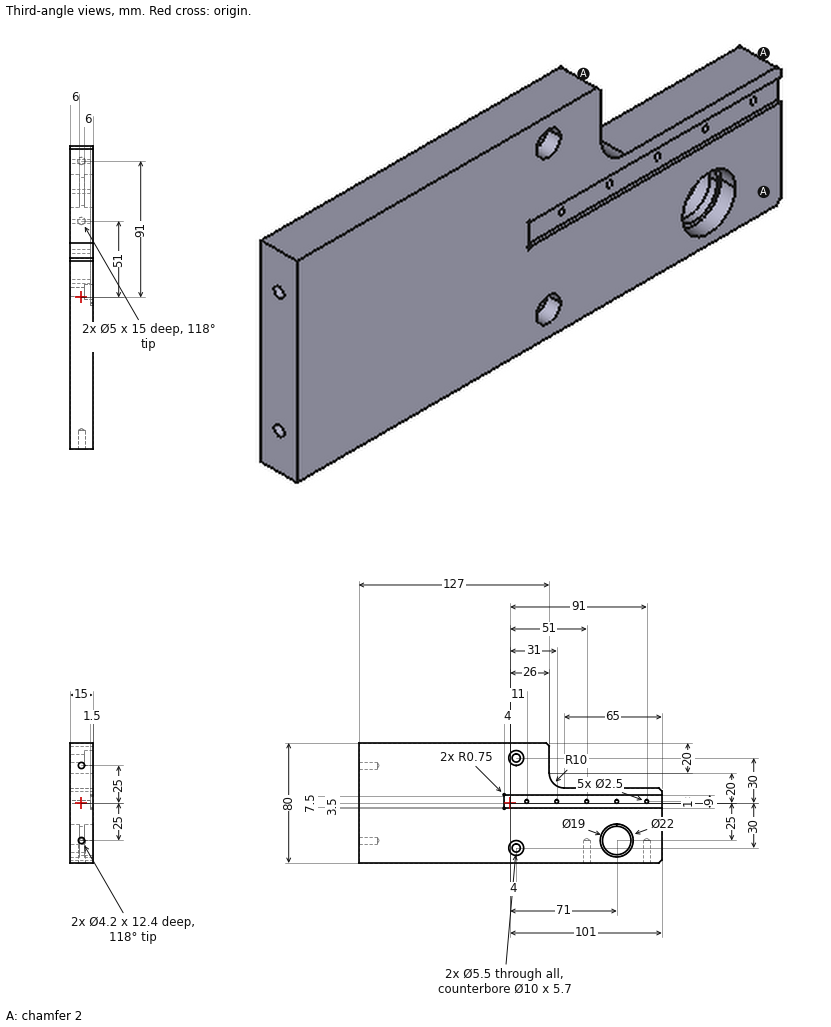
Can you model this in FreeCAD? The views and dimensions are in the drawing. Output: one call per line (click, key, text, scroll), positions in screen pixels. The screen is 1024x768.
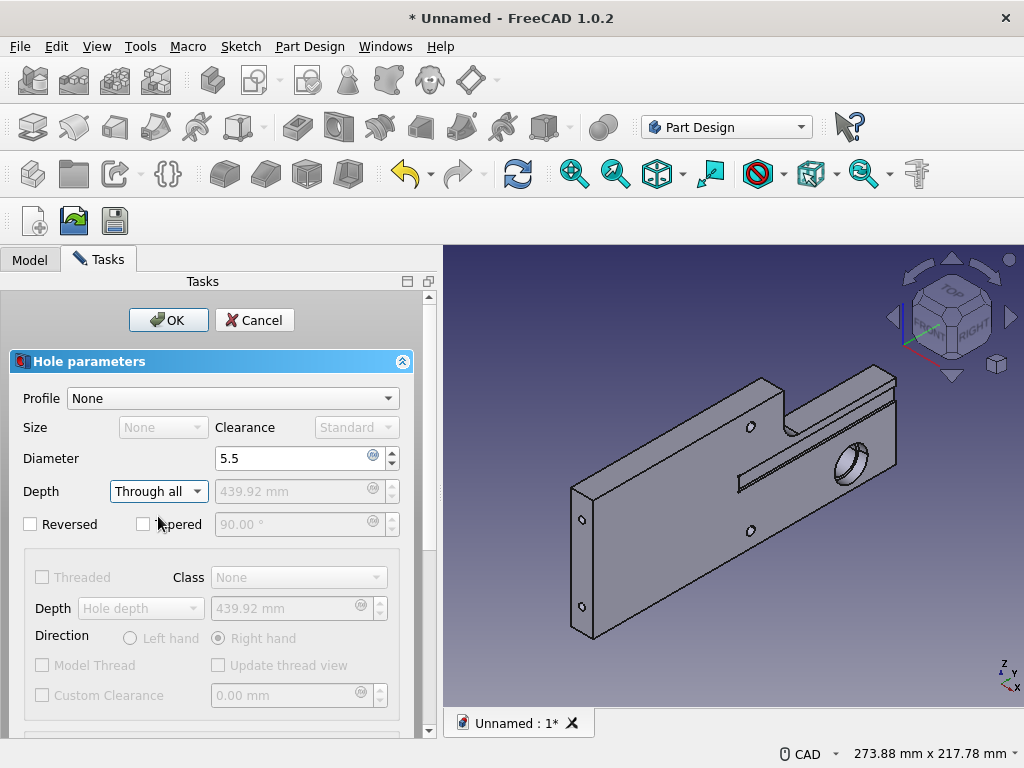
scroll(429, 514, down, 2)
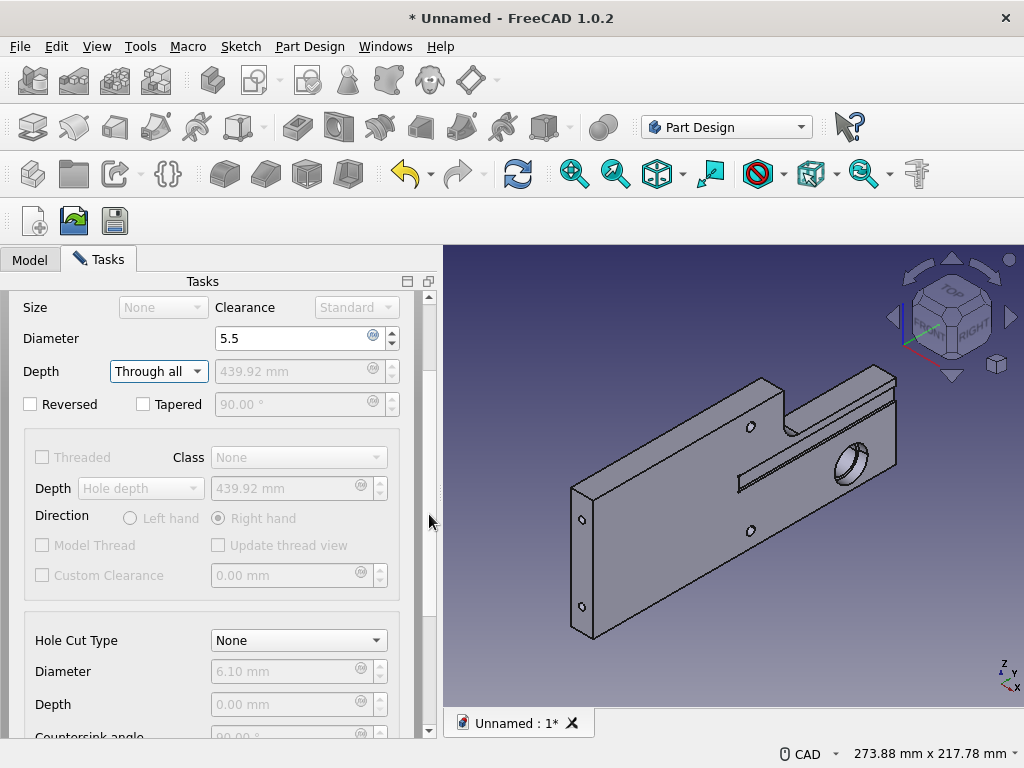
click(300, 640)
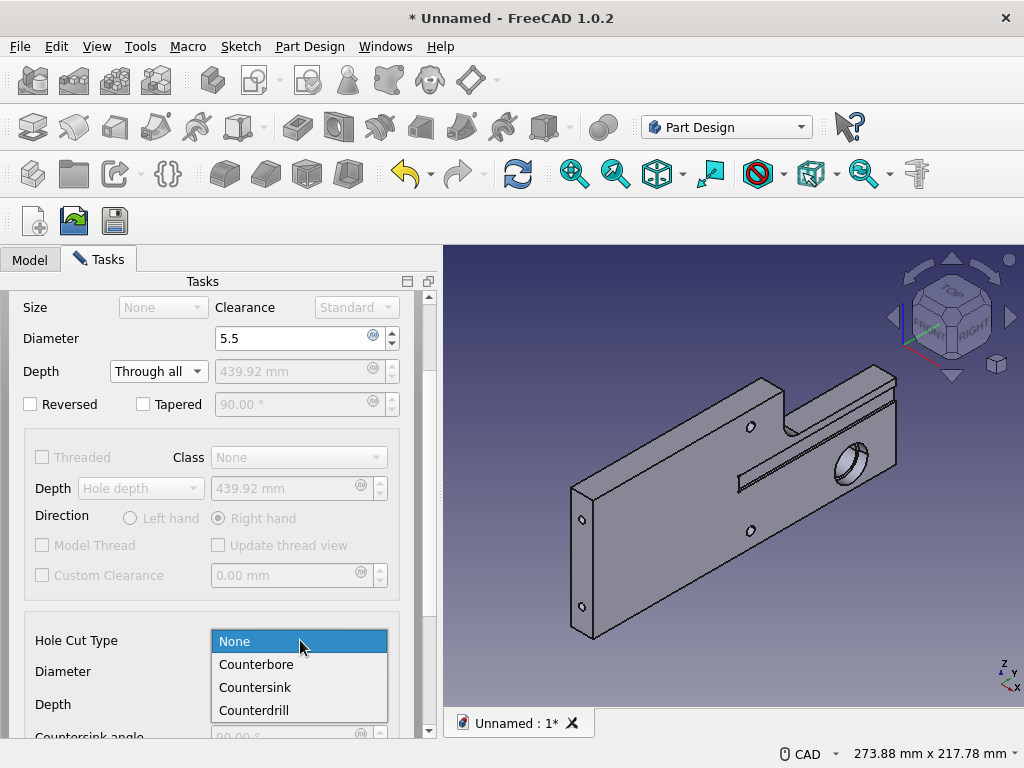
click(298, 664)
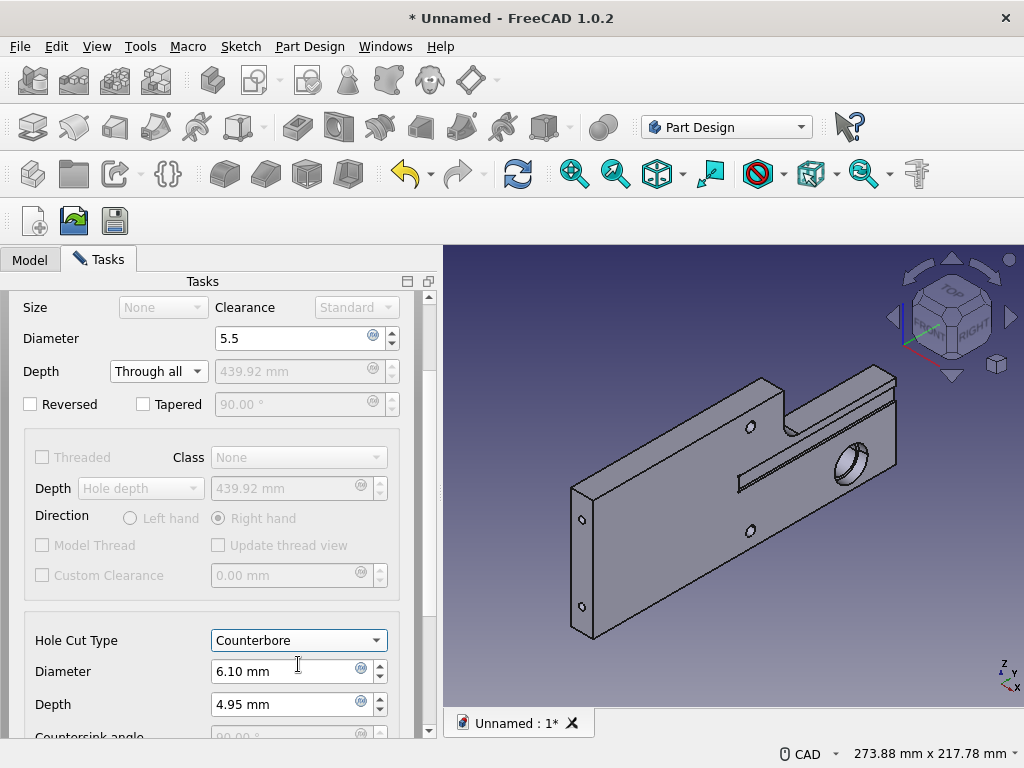
triple_click(292, 672)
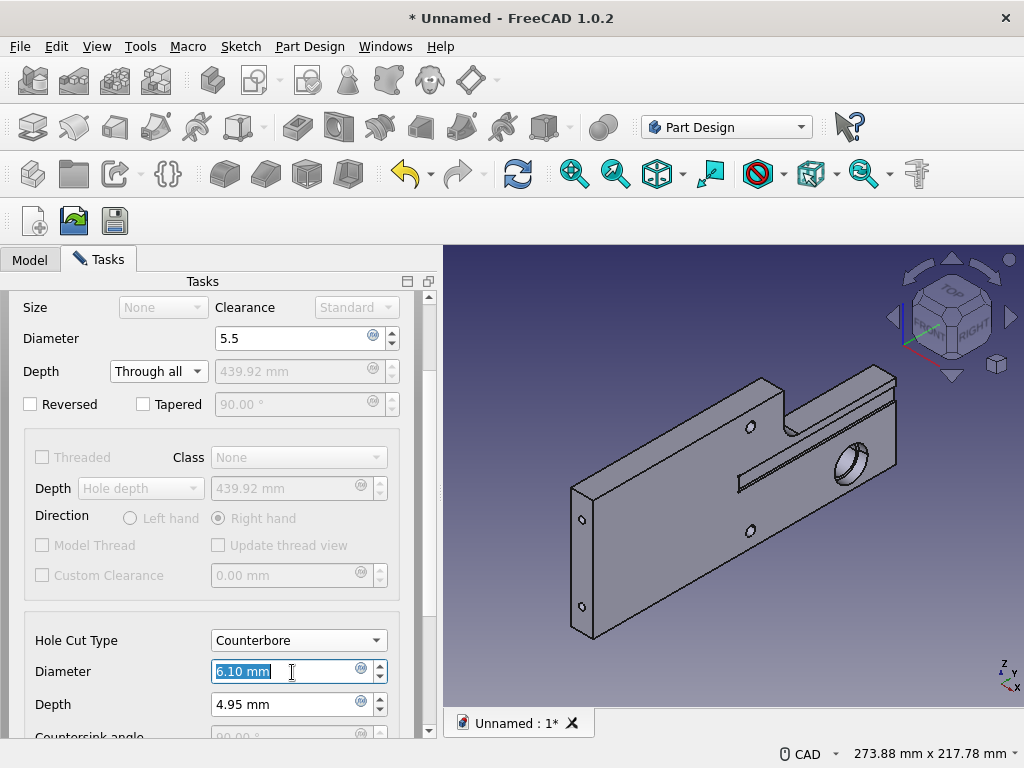
text(10)
key(Tab)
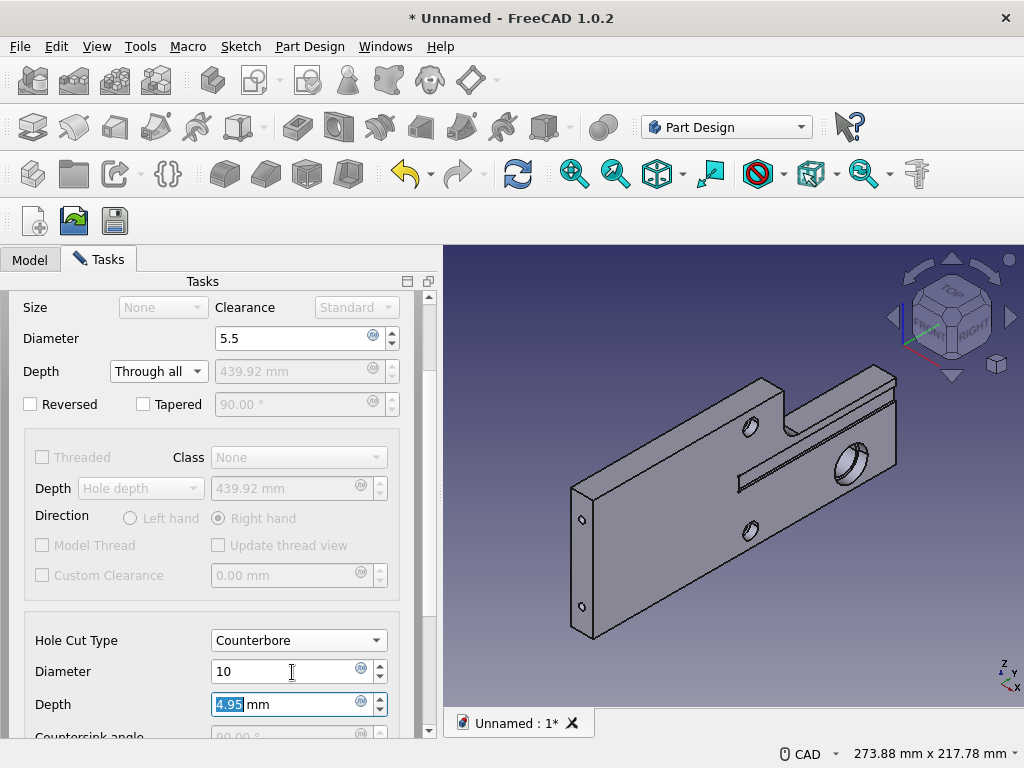
text(5.7)
key(Tab)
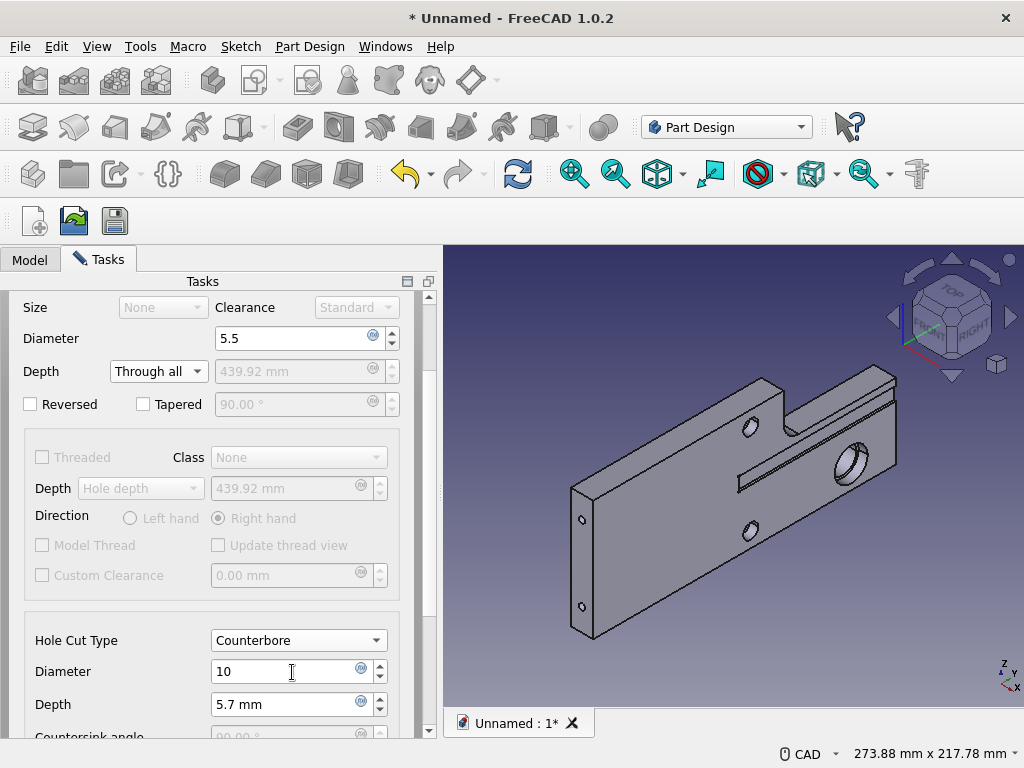
scroll(429, 514, up, 3)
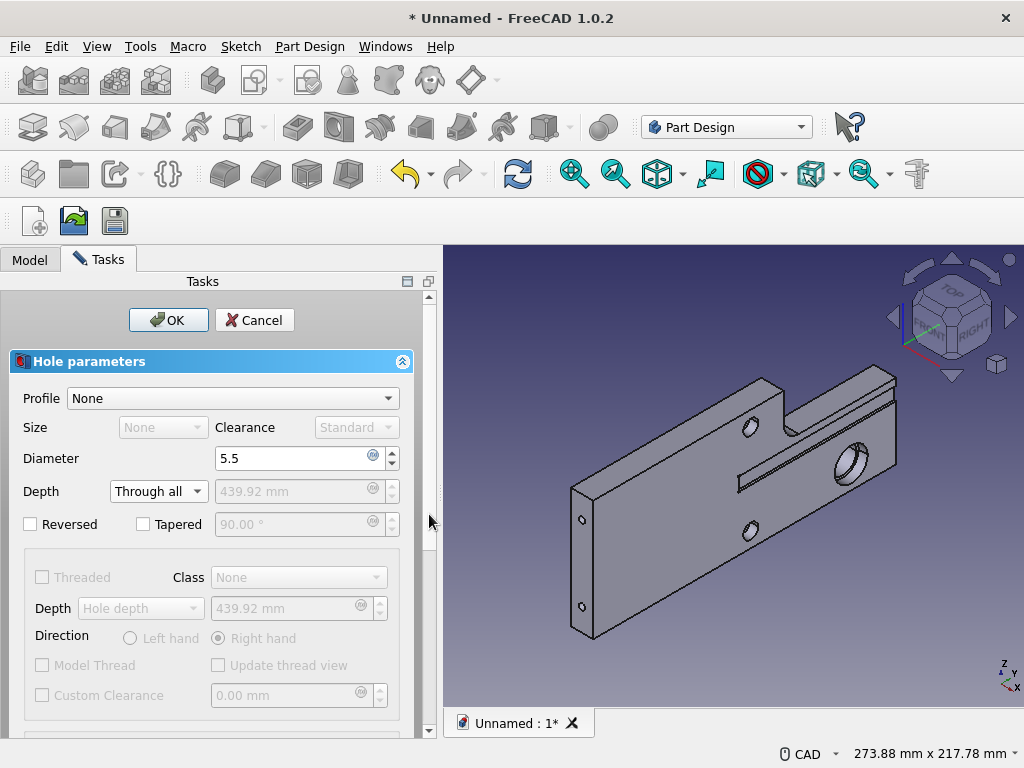
click(169, 320)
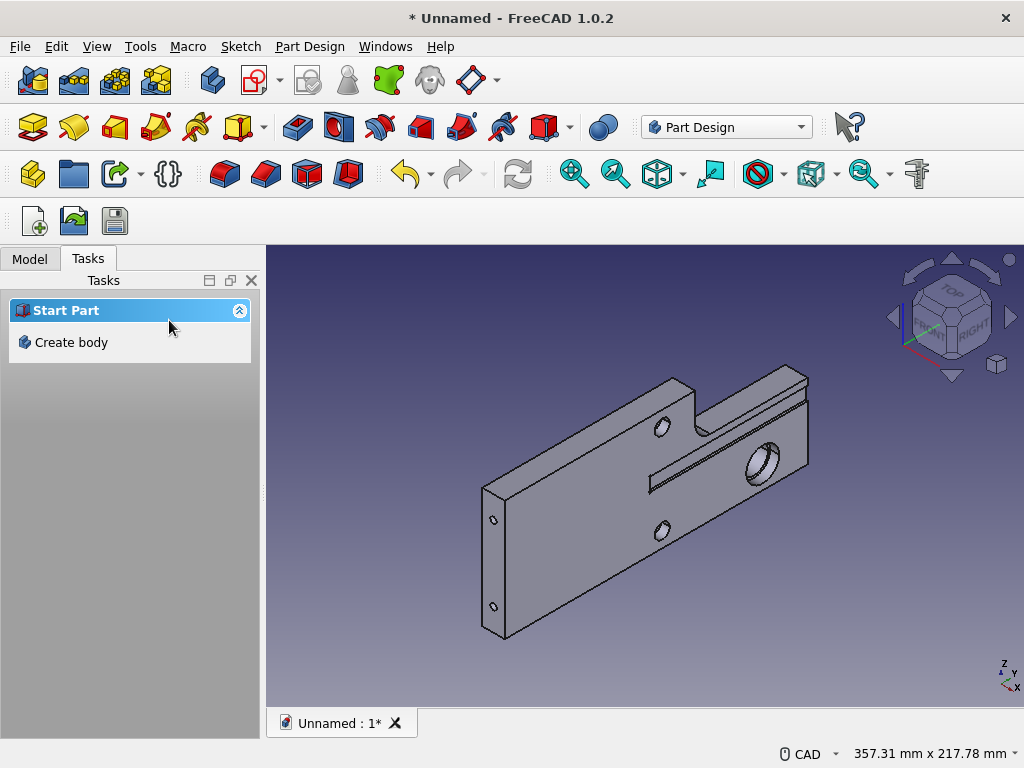
key(3)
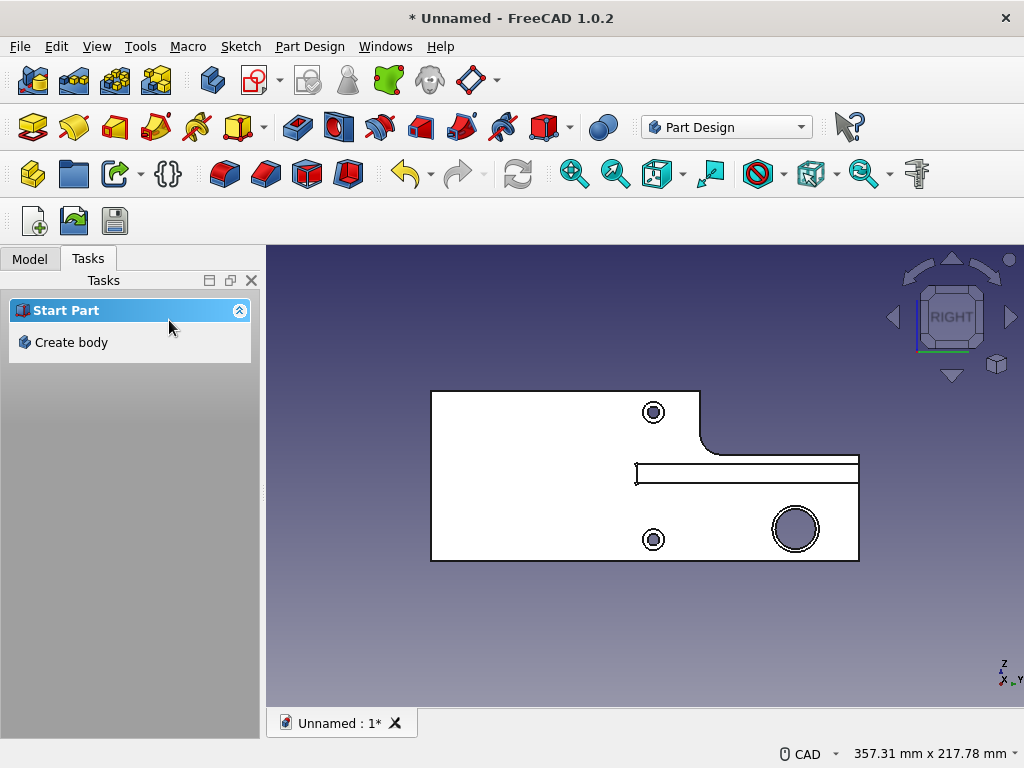
click(843, 473)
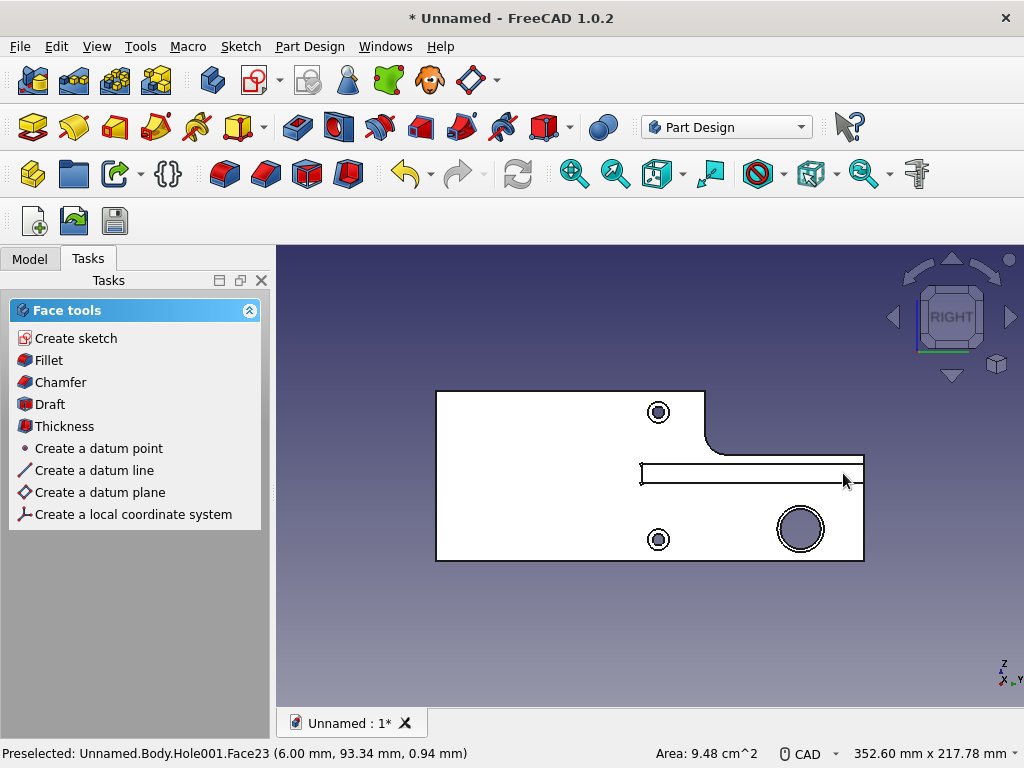
click(254, 80)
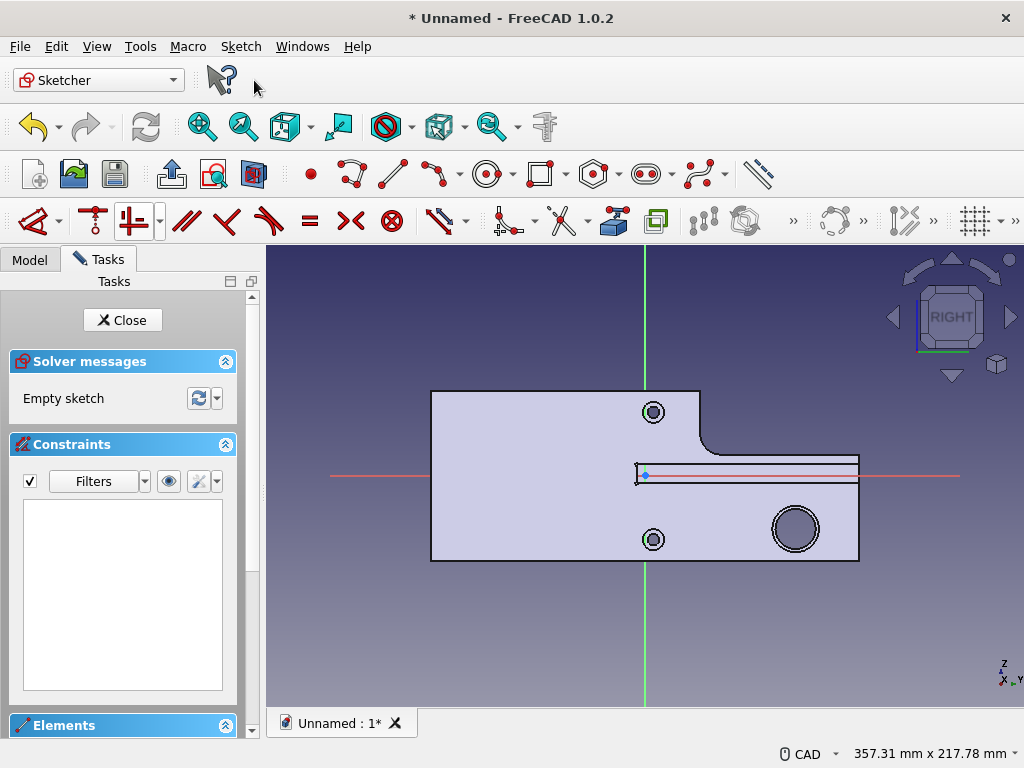
scroll(859, 472, up, 4)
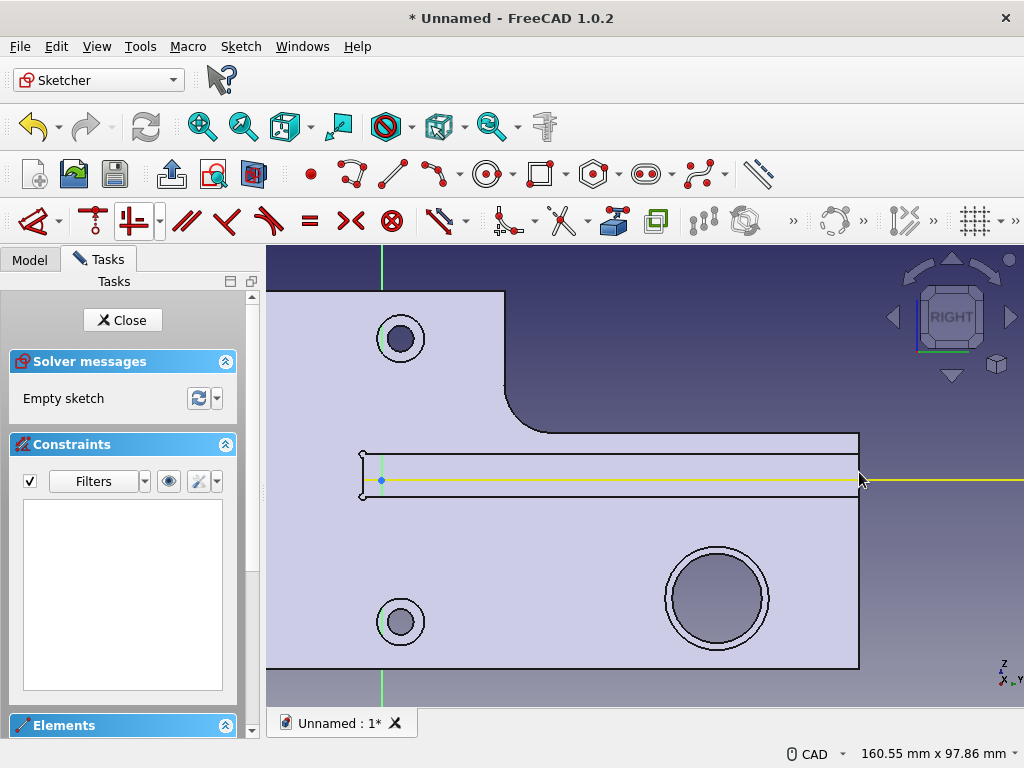
key(g)
key(c)